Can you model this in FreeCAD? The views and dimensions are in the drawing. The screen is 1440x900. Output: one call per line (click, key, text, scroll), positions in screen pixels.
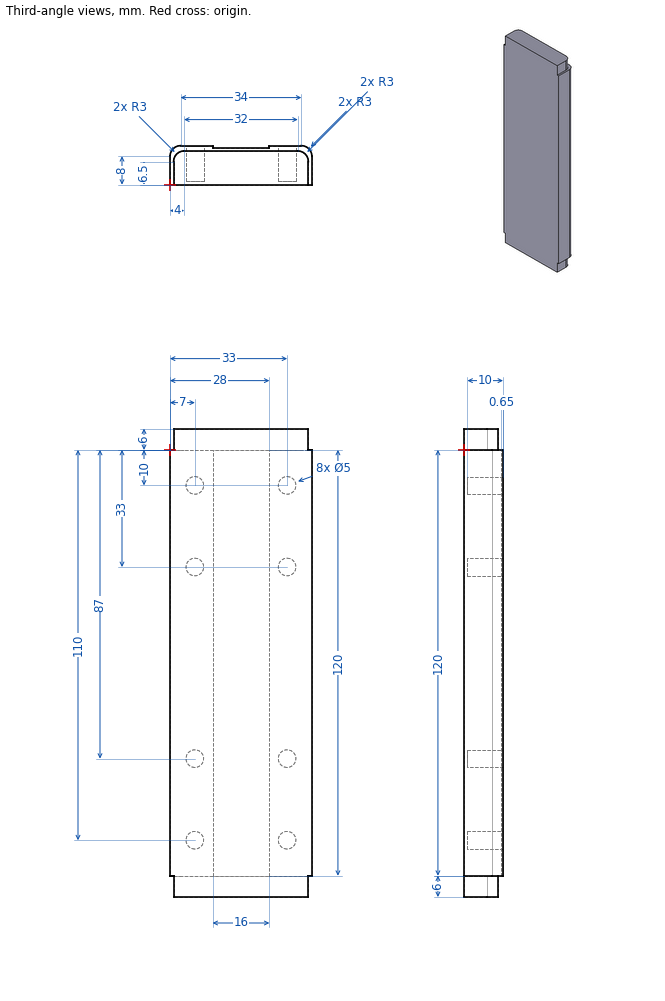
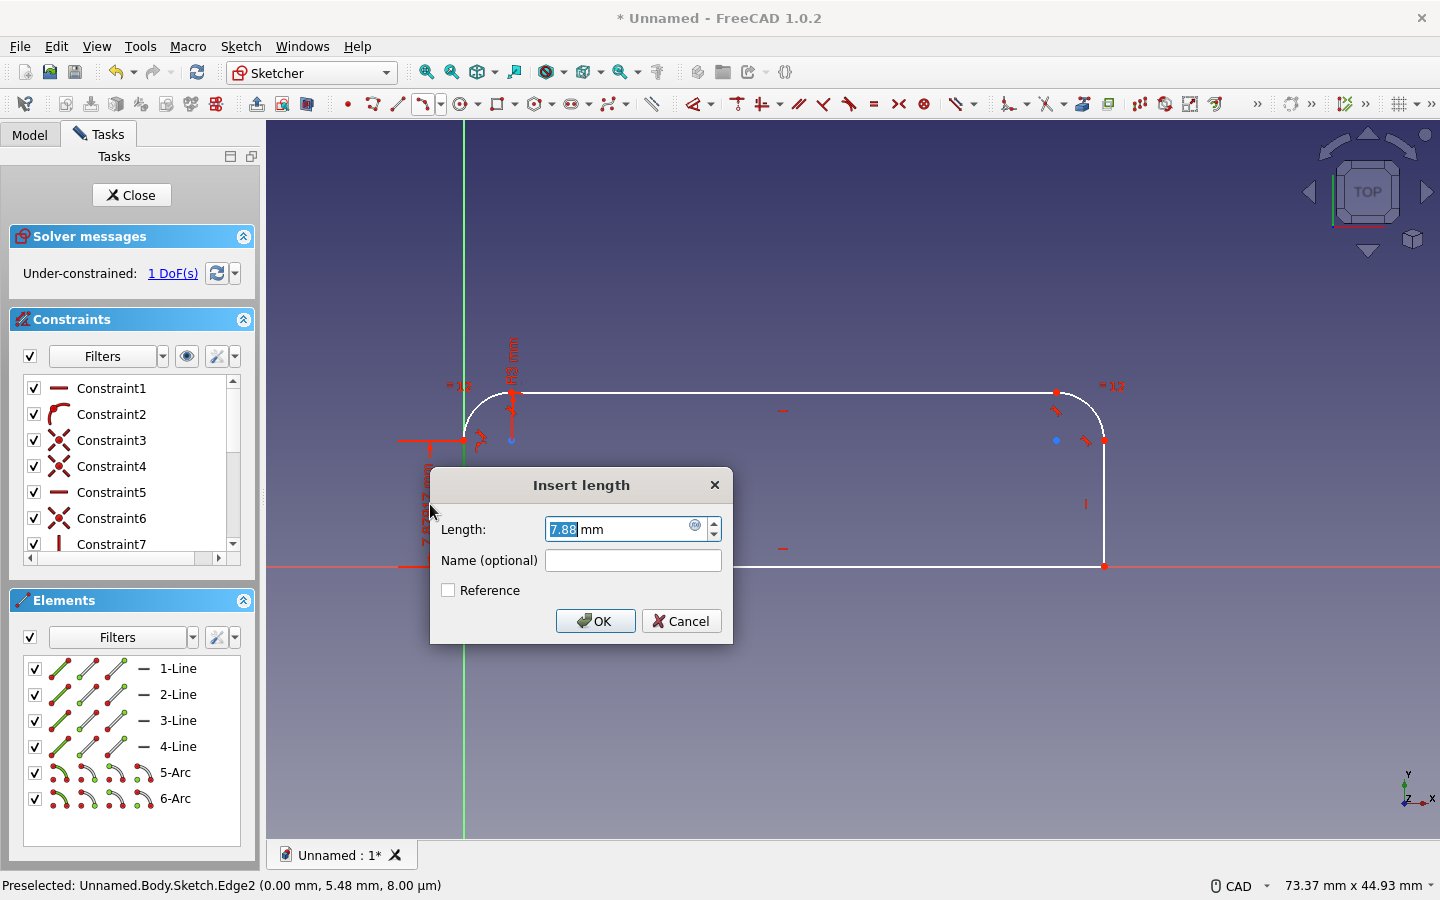
text(8)
key(Return)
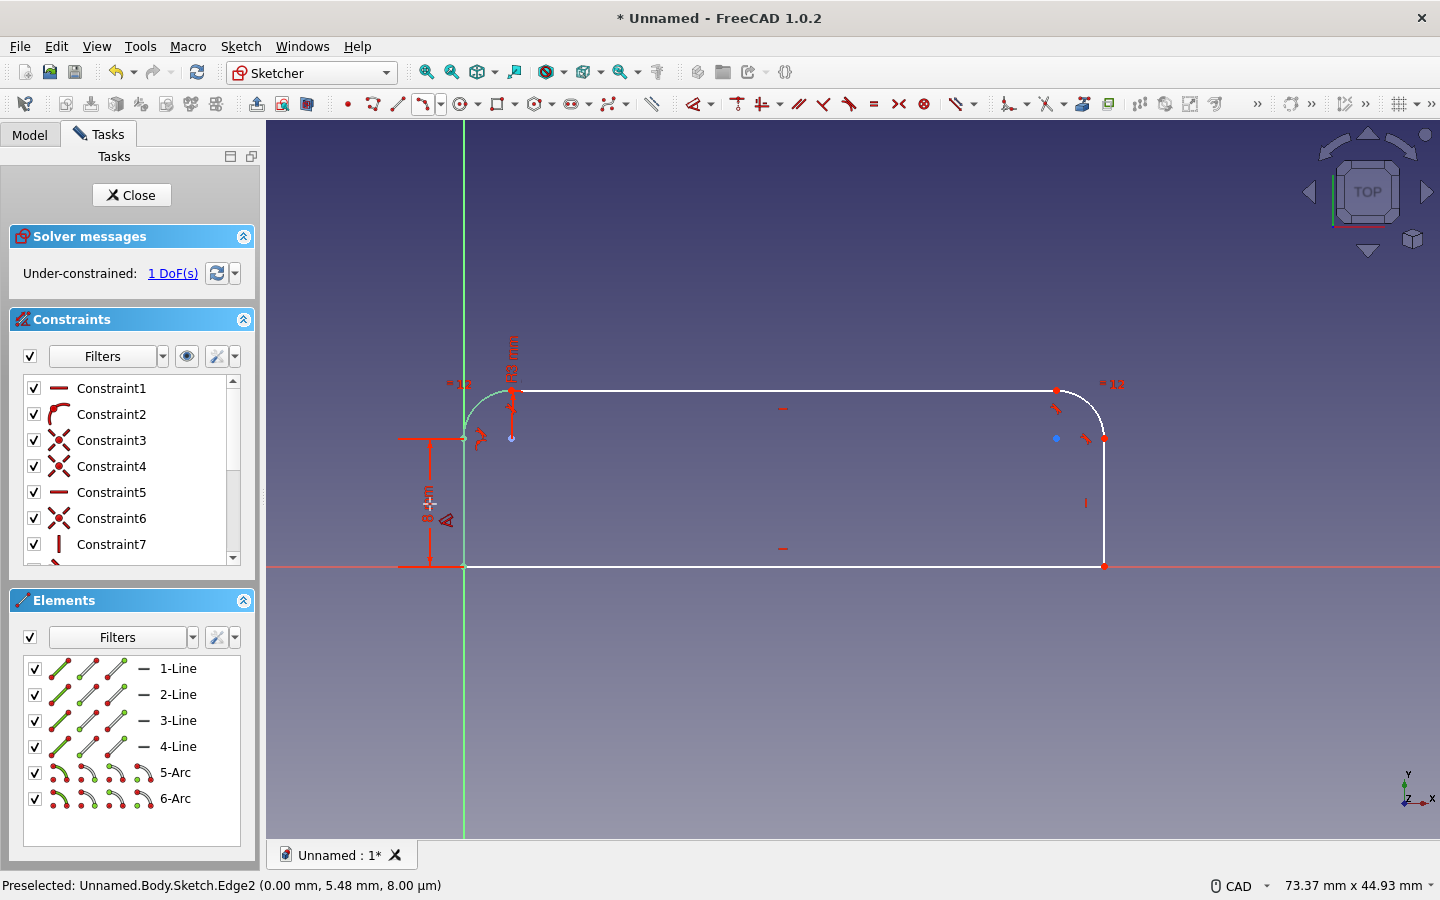
click(893, 391)
click(784, 357)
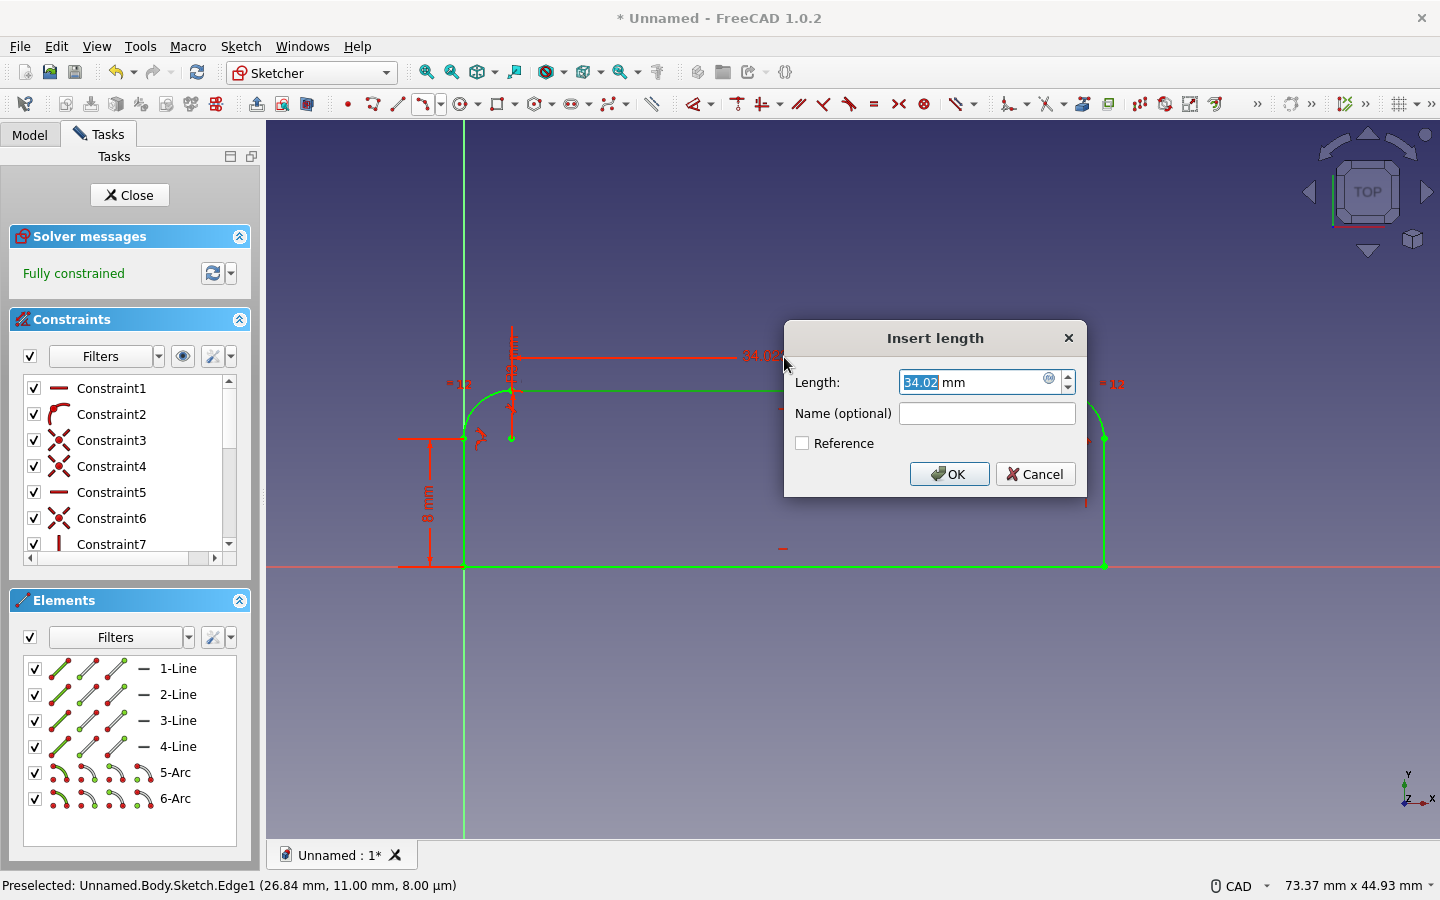
text(34)
key(Return)
key(Escape)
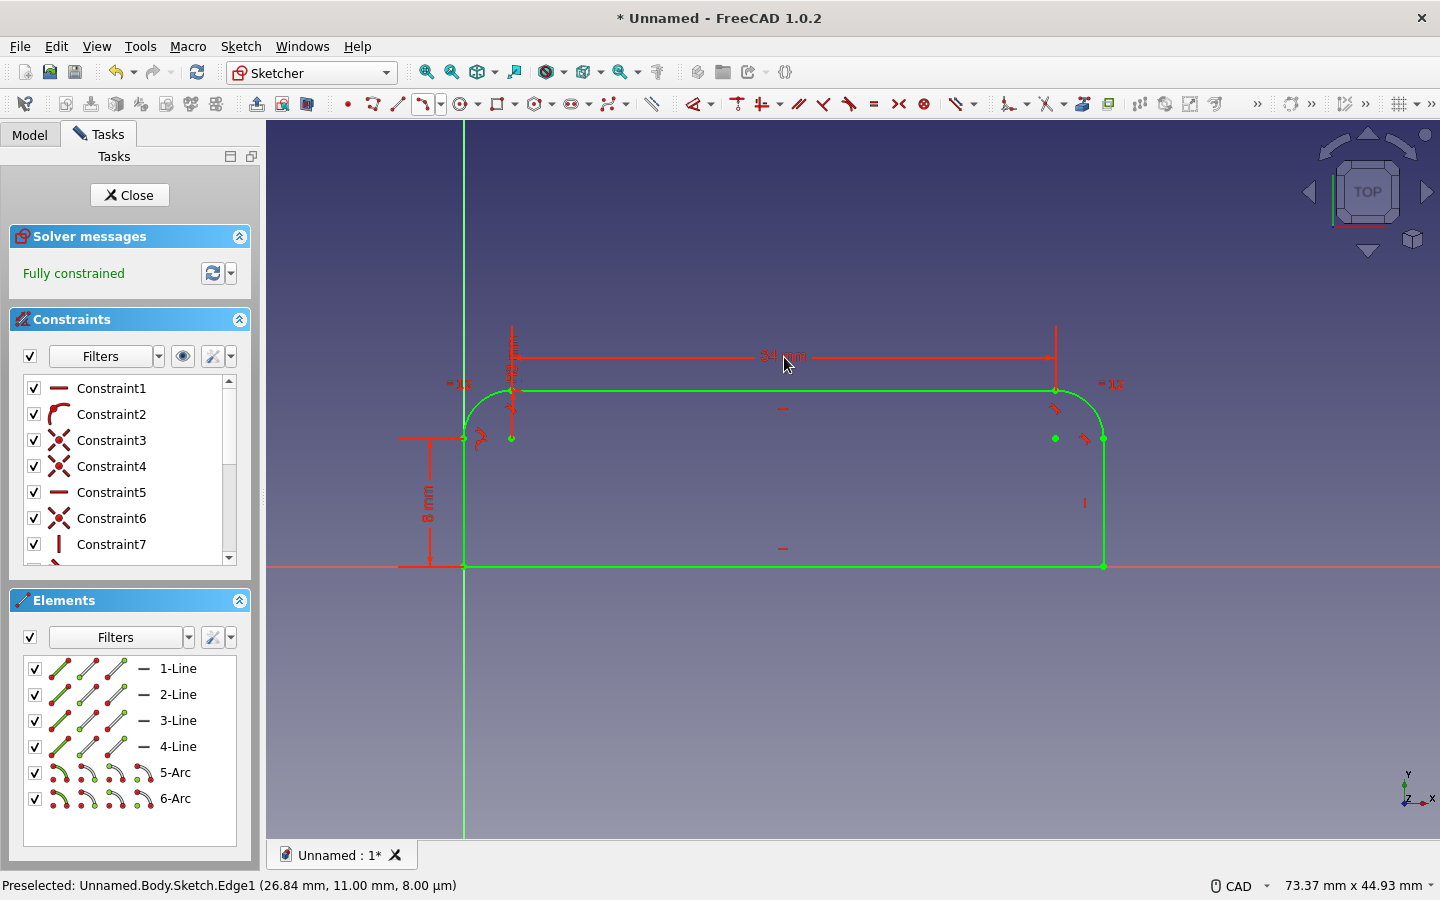
click(130, 195)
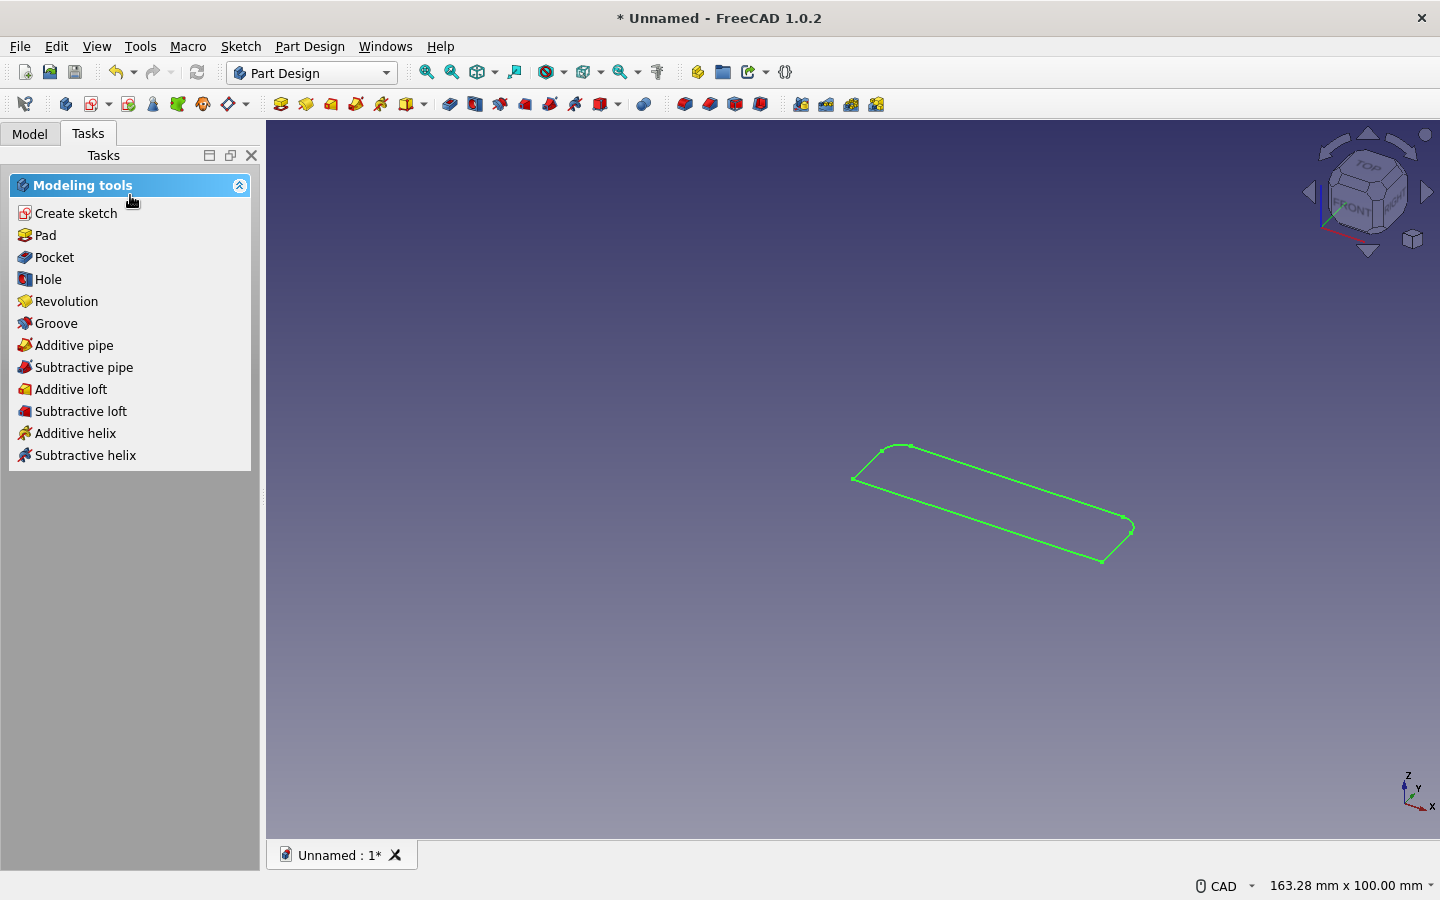
click(281, 104)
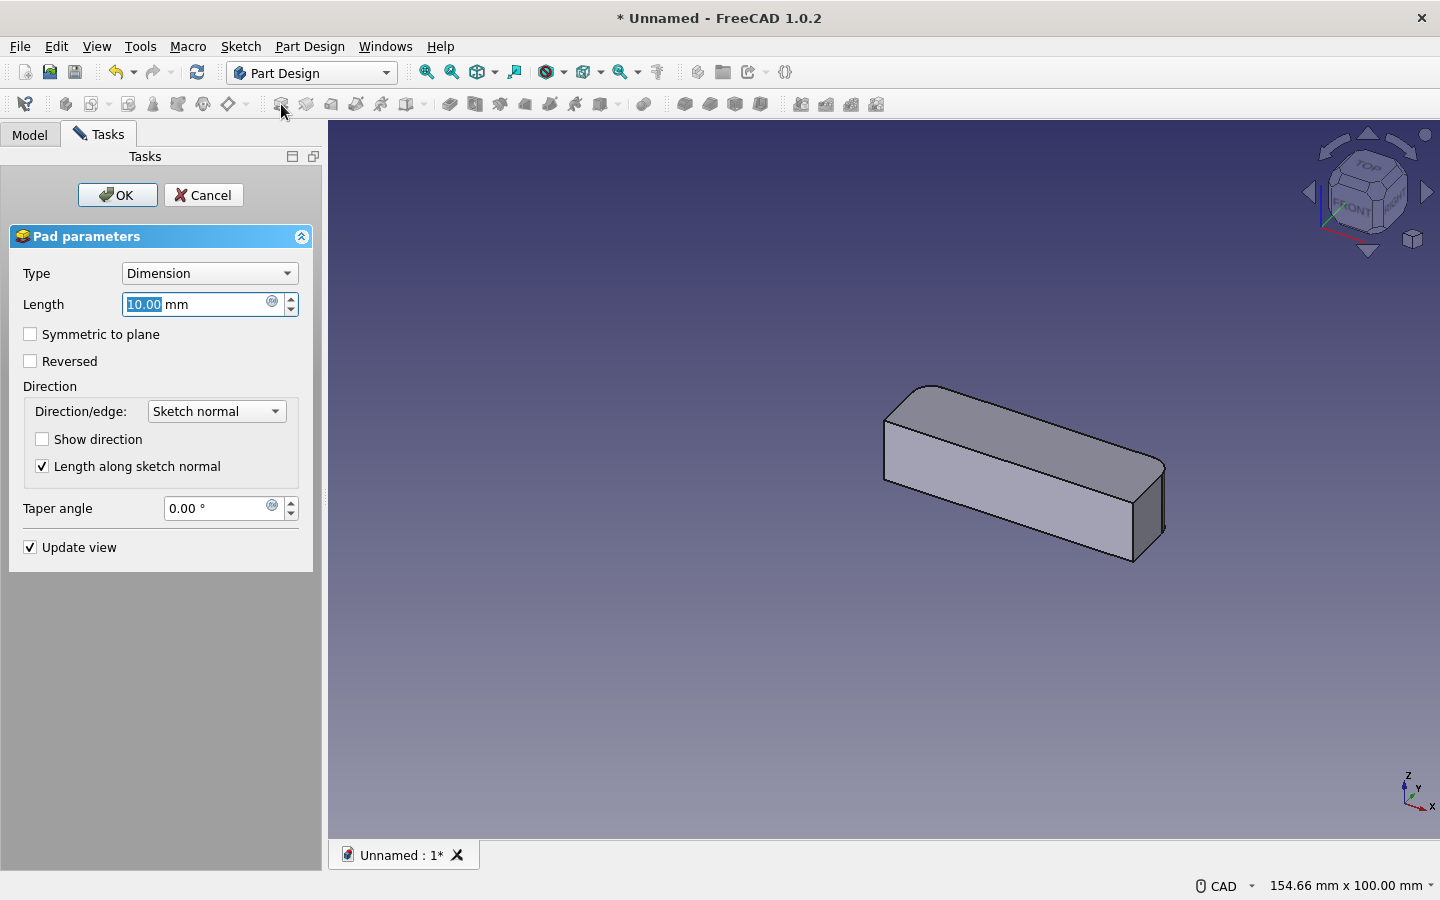
text(120)
key(Tab)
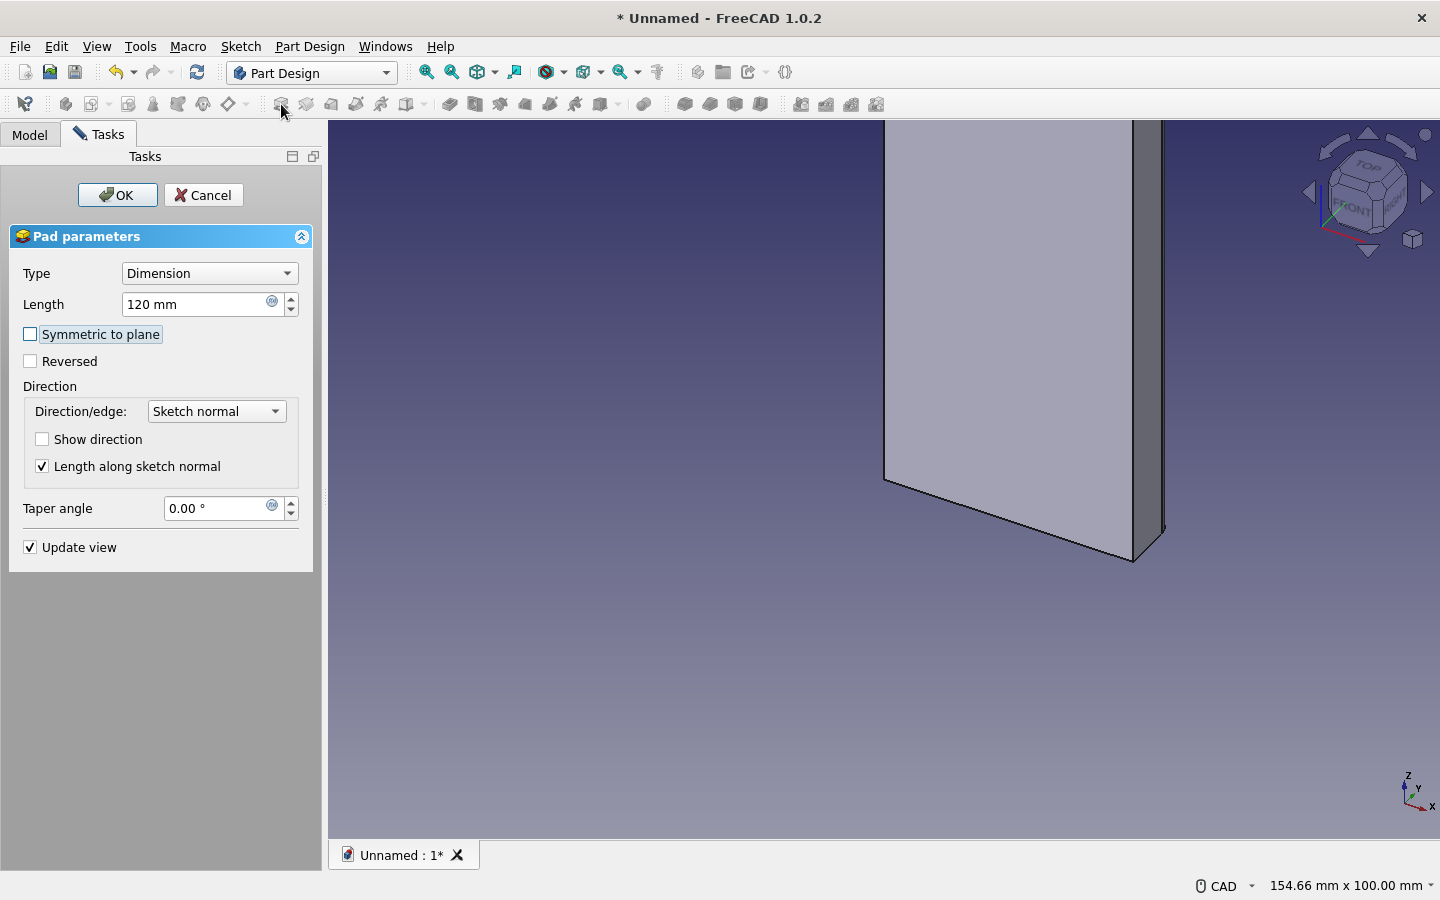
click(31, 361)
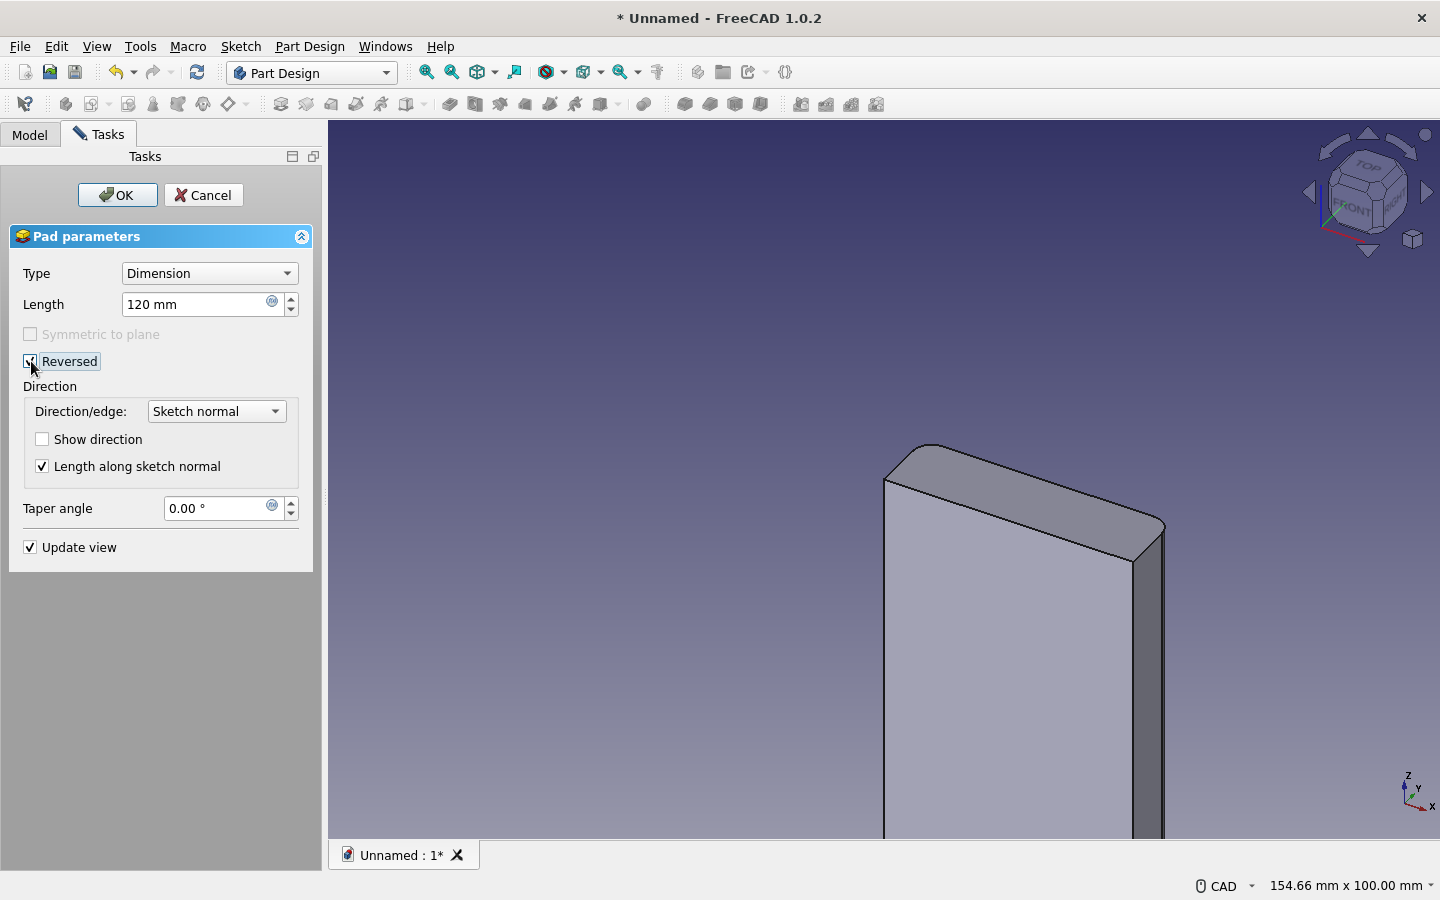
click(118, 195)